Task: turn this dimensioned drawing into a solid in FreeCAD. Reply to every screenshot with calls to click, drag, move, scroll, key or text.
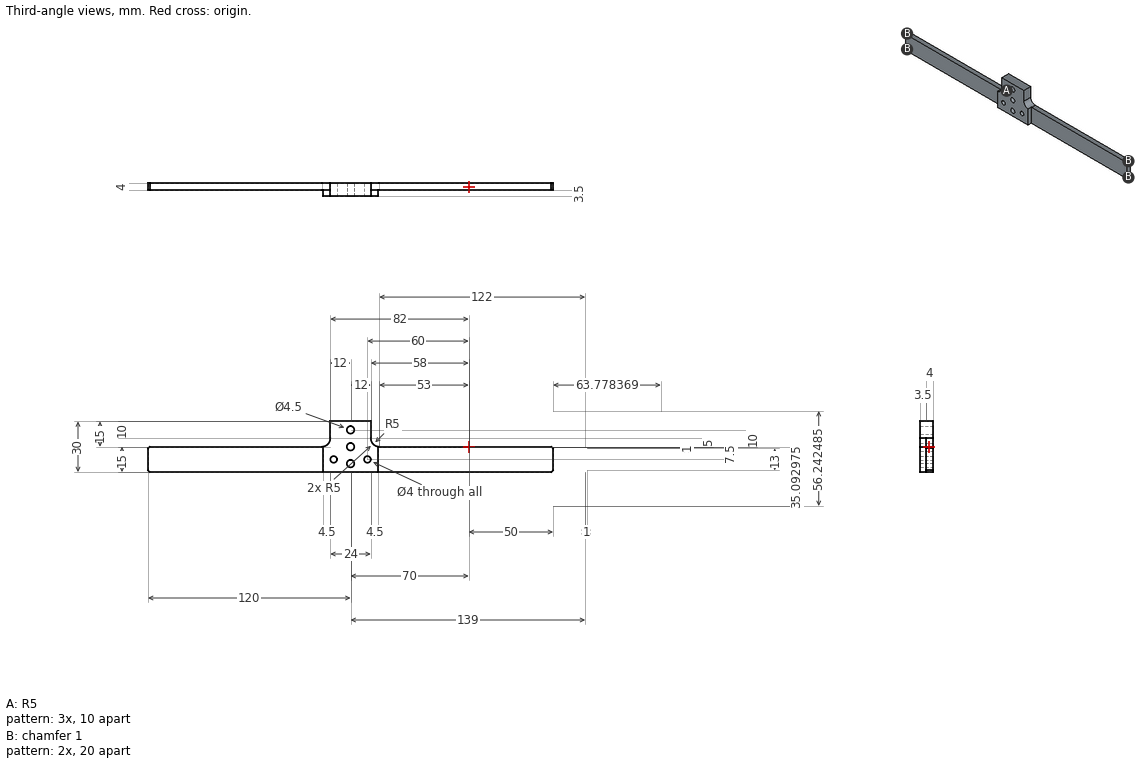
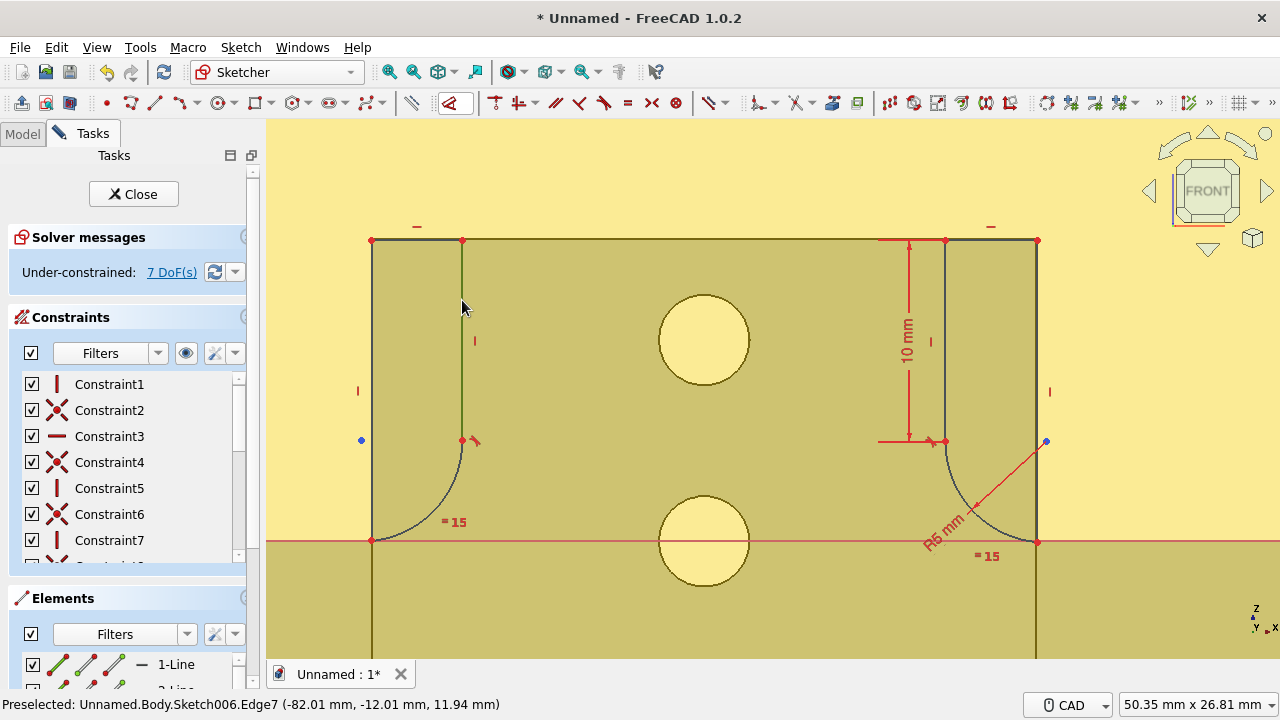
click(468, 104)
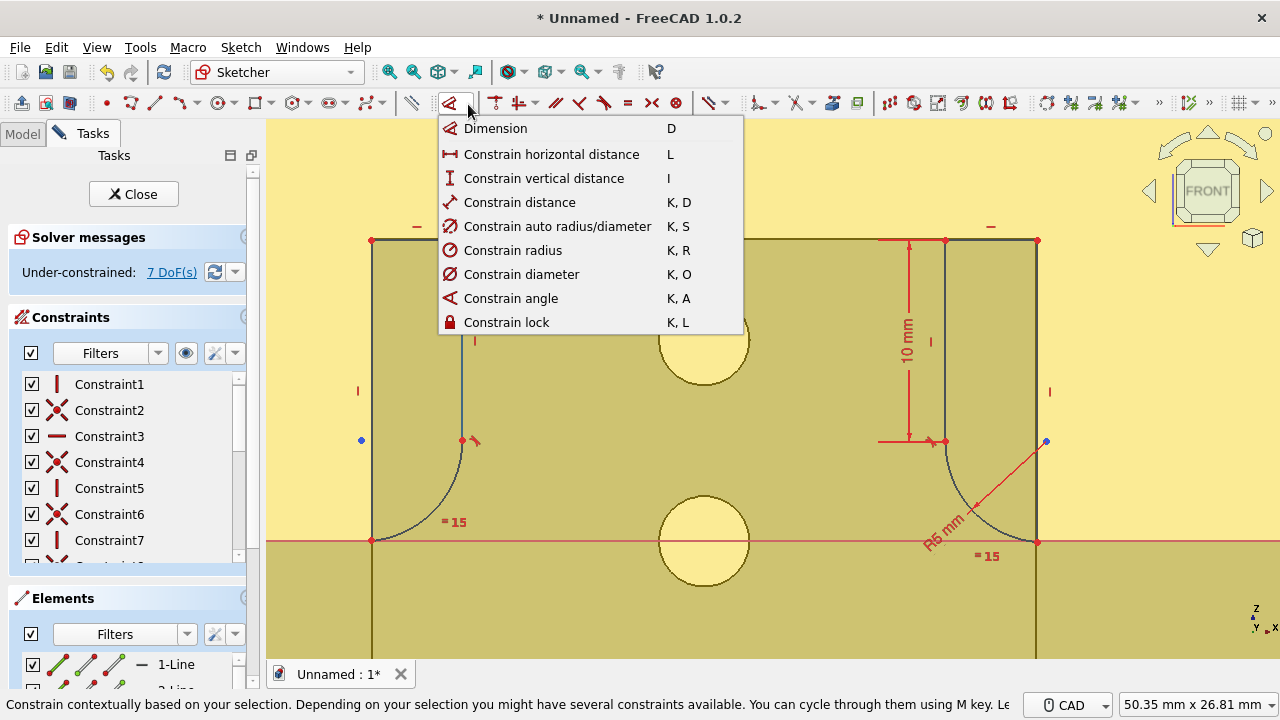
click(591, 178)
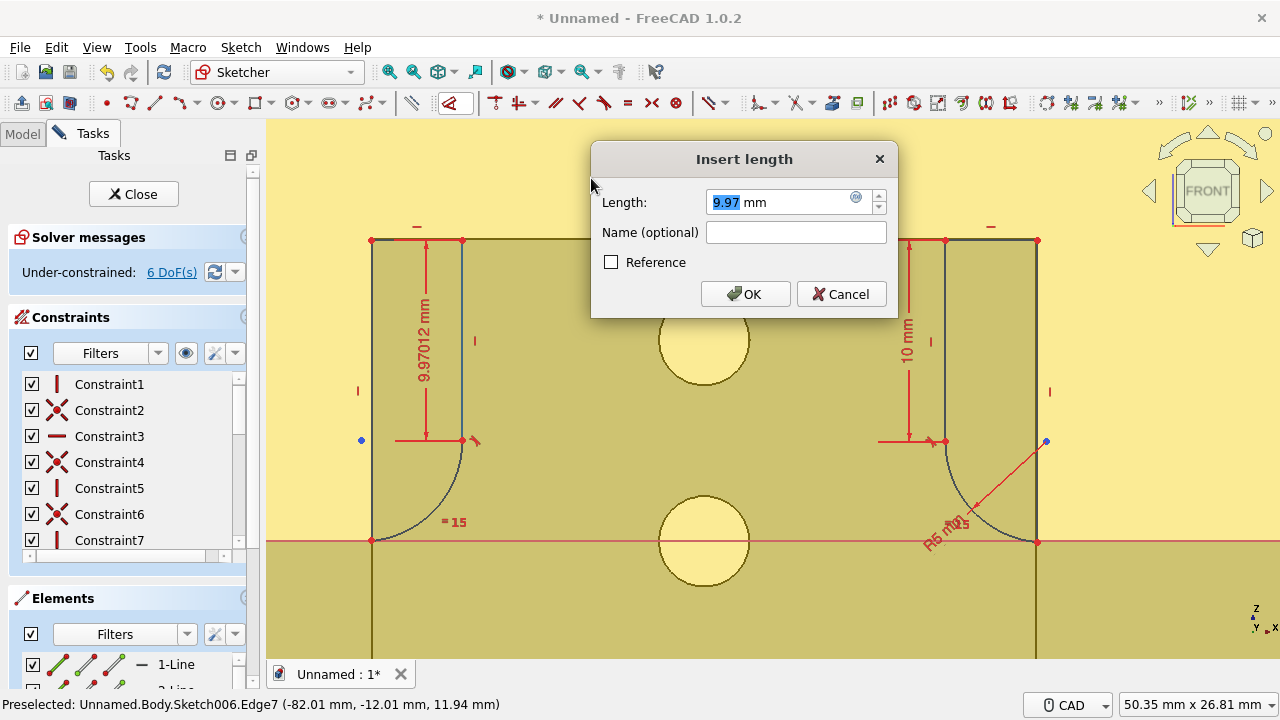
text(10)
key(Return)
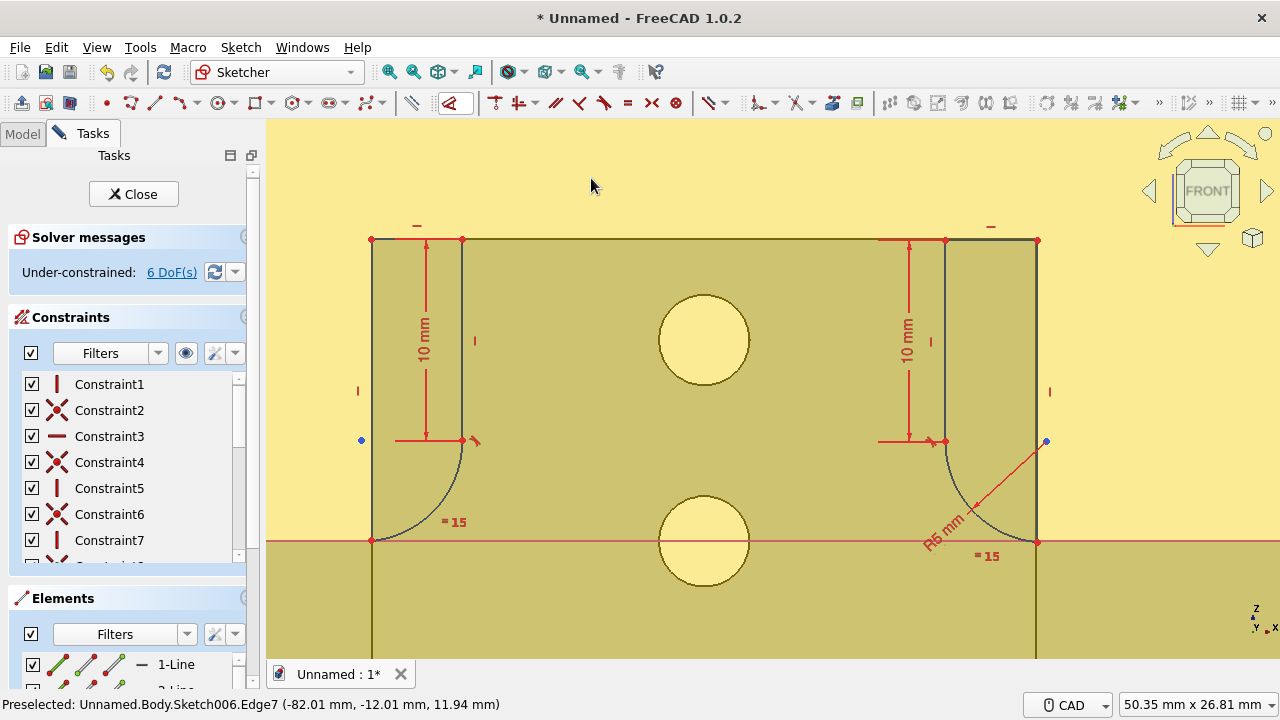
click(945, 442)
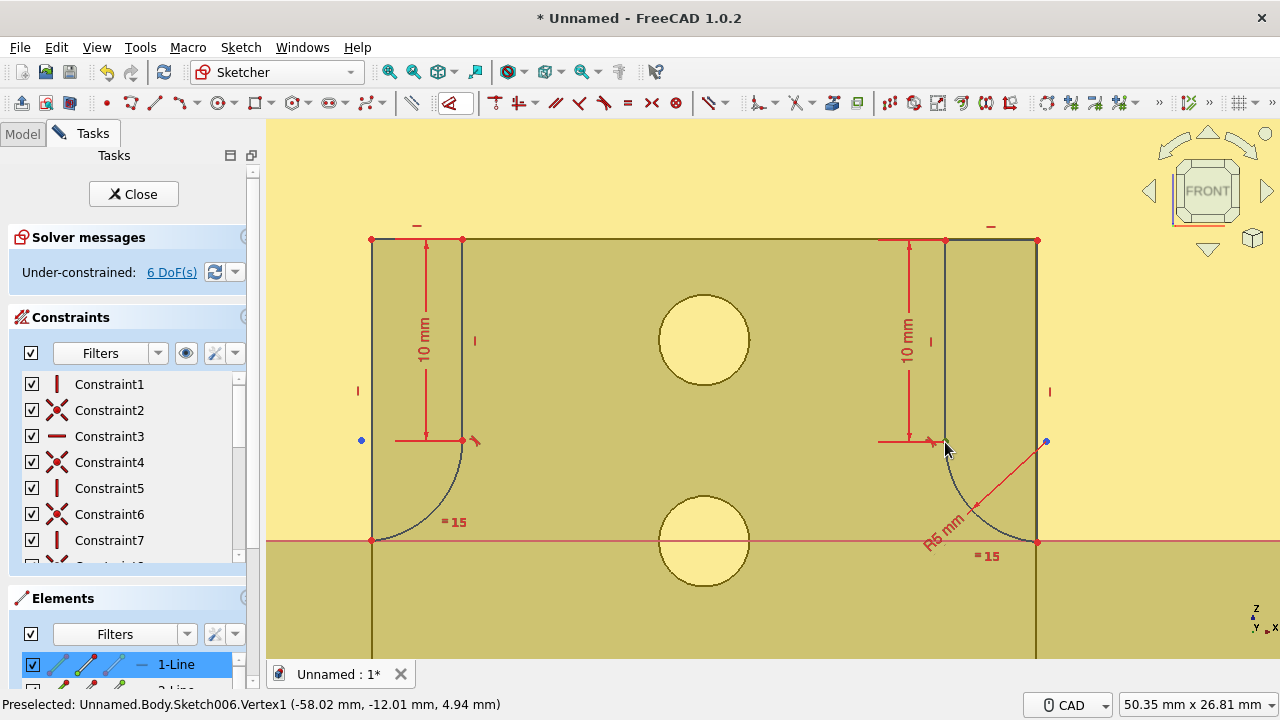
click(468, 104)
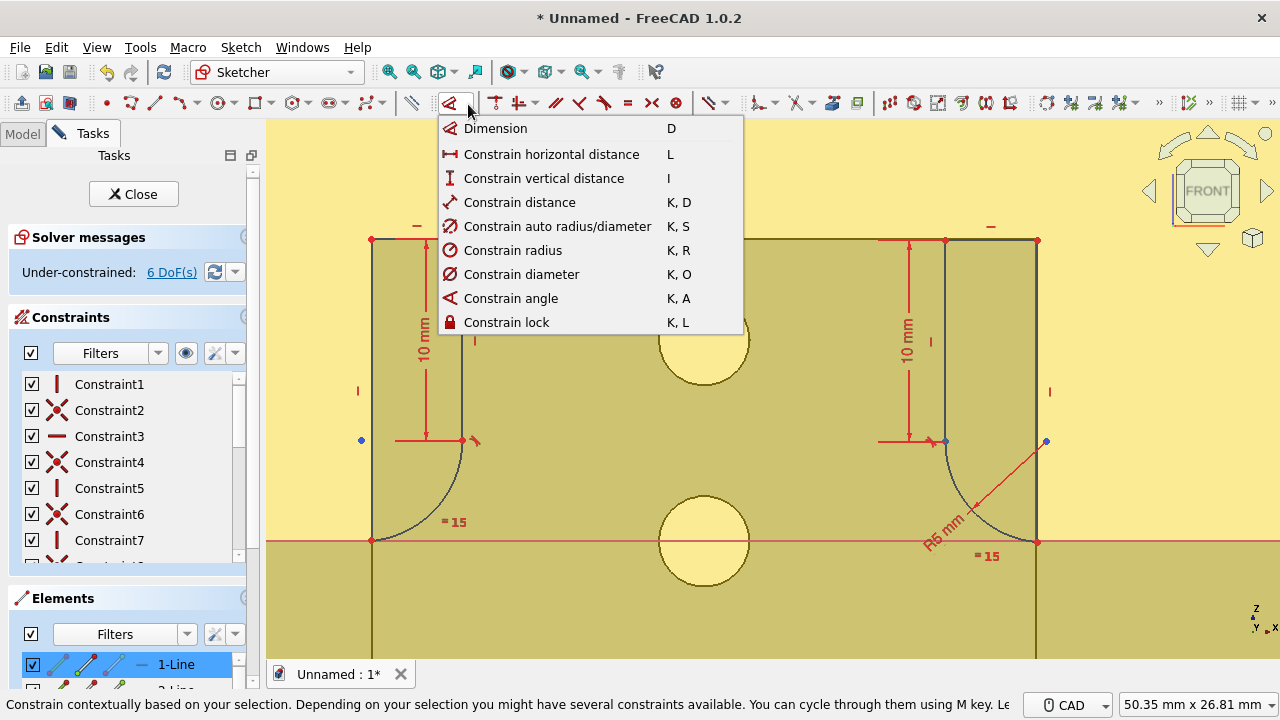
click(591, 178)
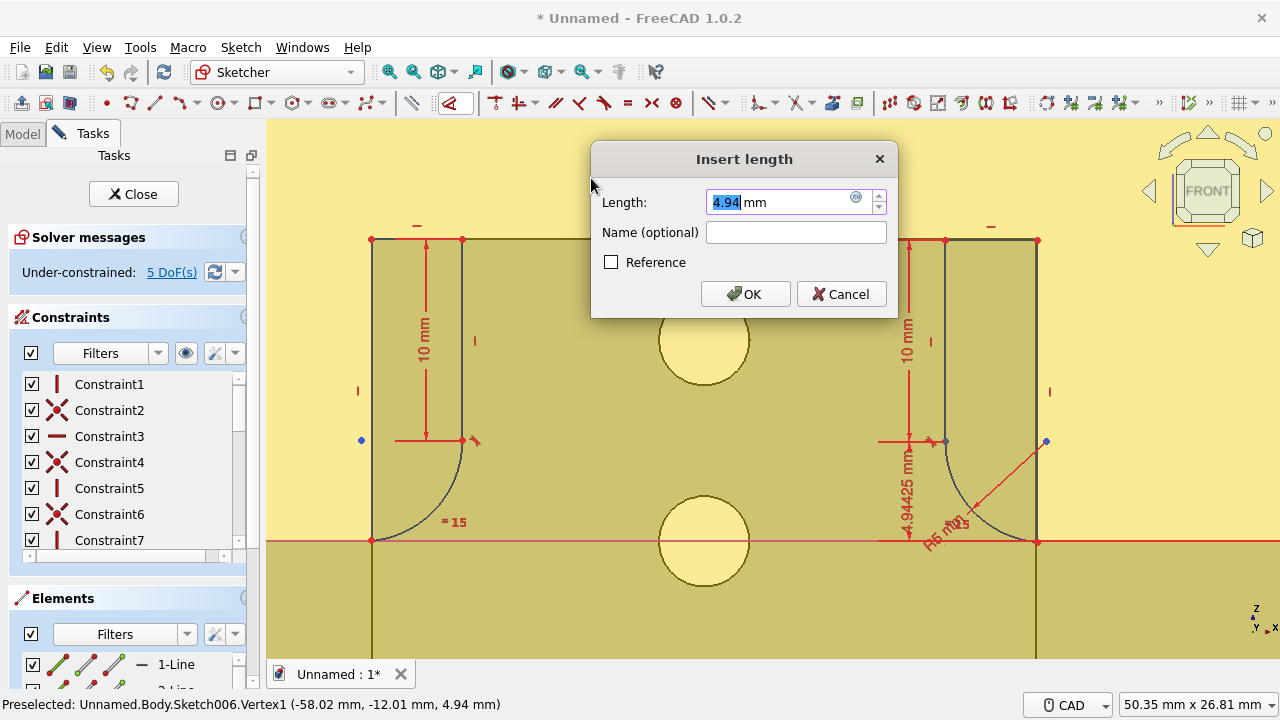
text(5)
key(Return)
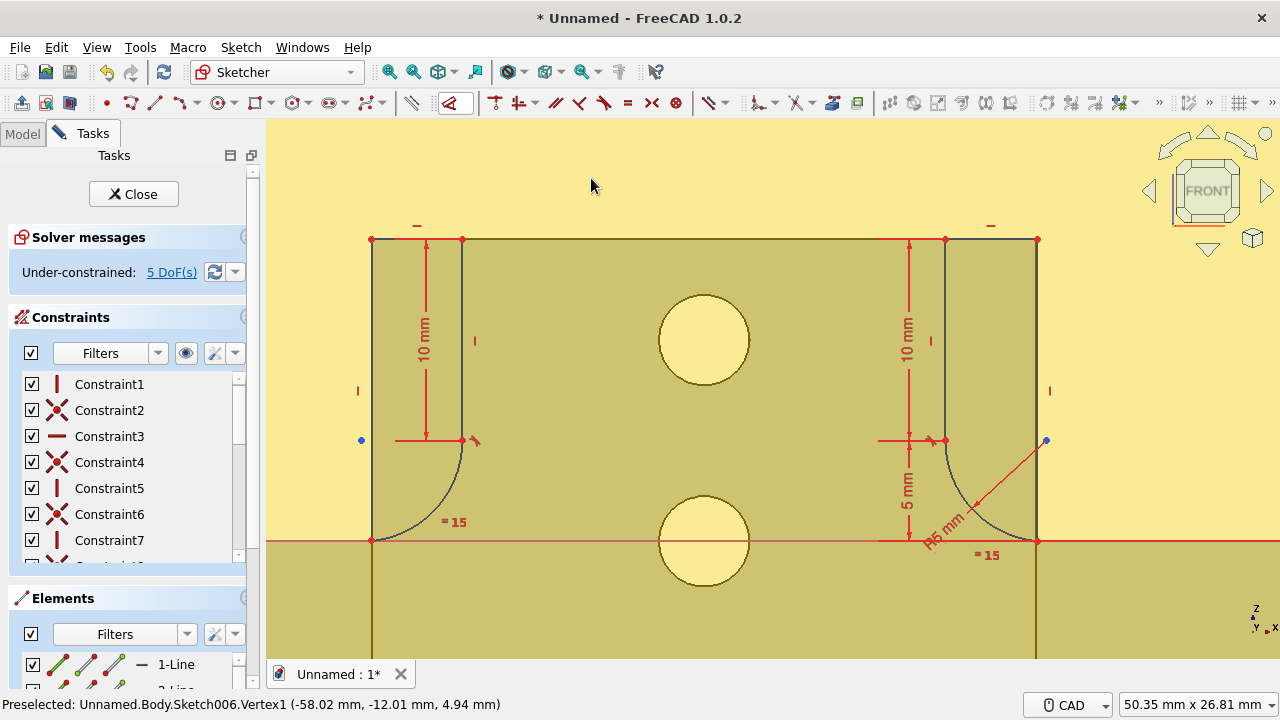
click(462, 441)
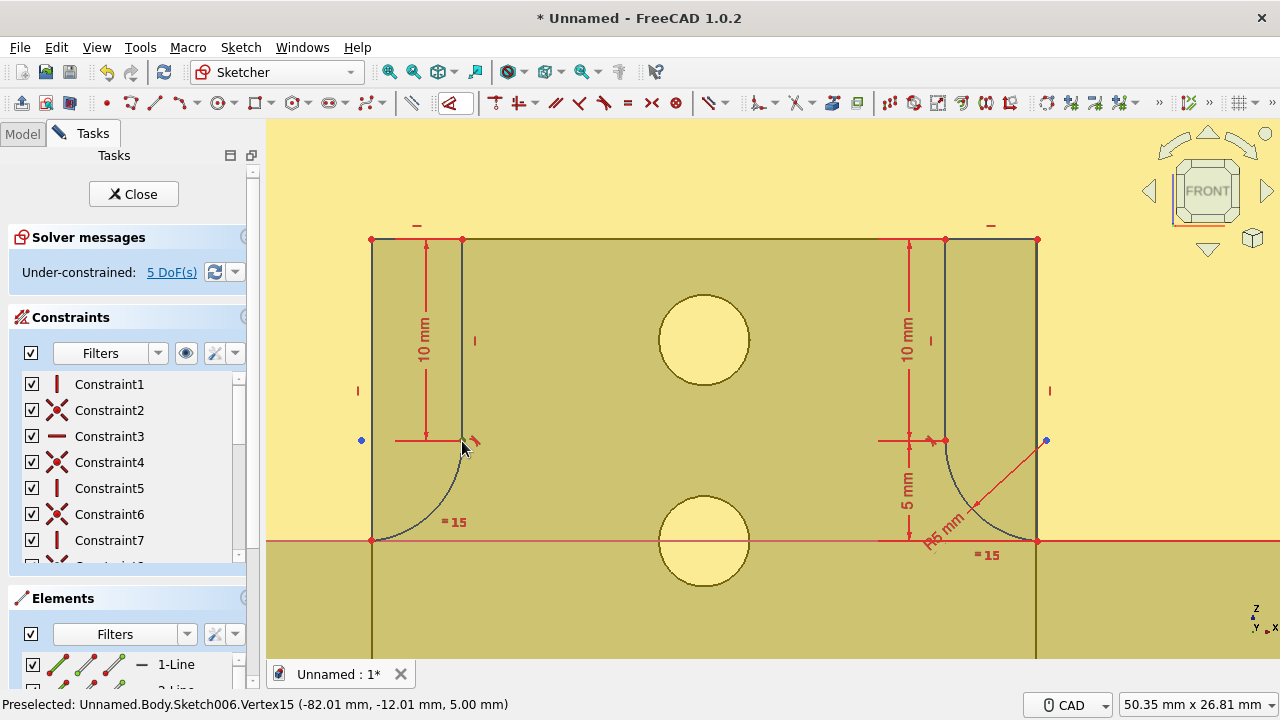
click(468, 104)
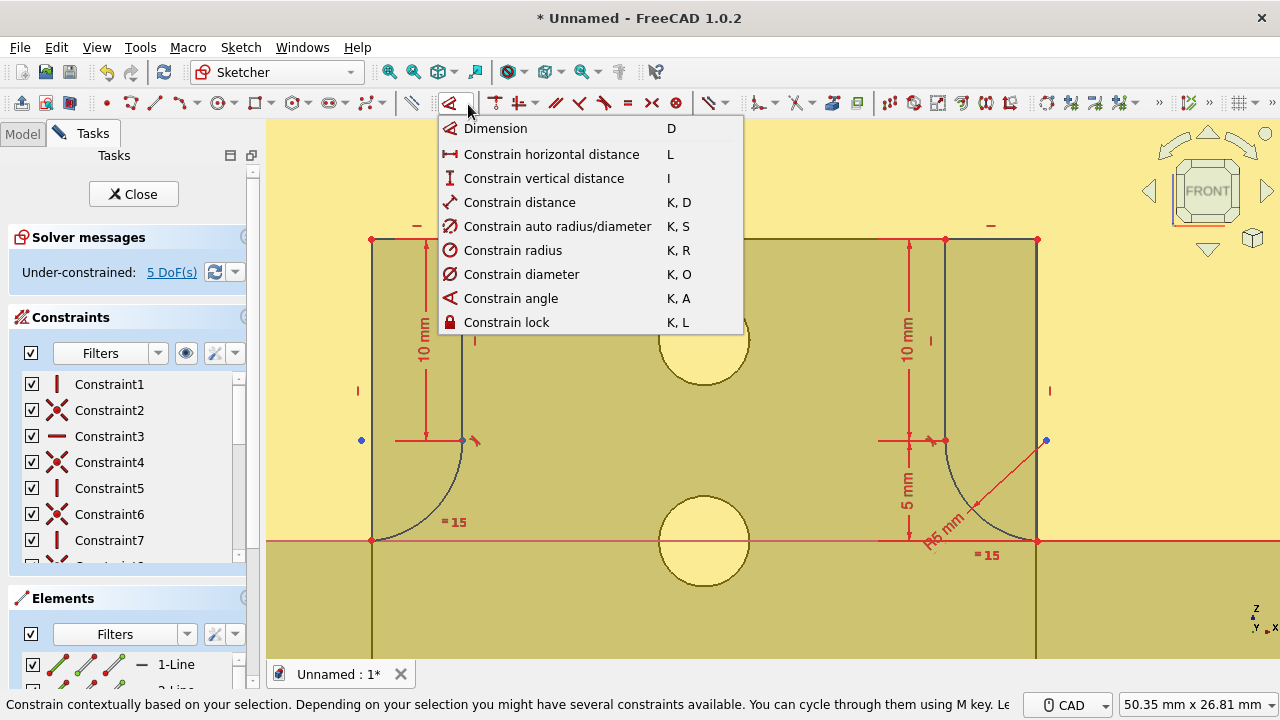
click(591, 178)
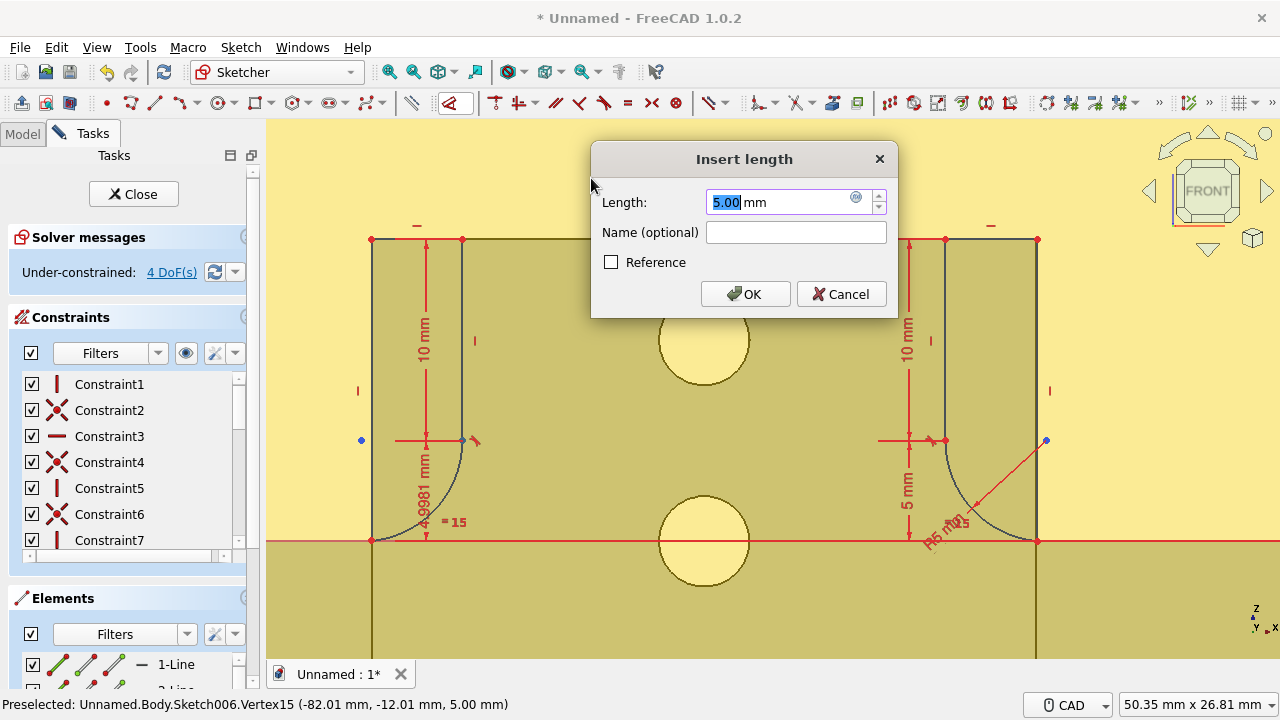
text(5)
key(Return)